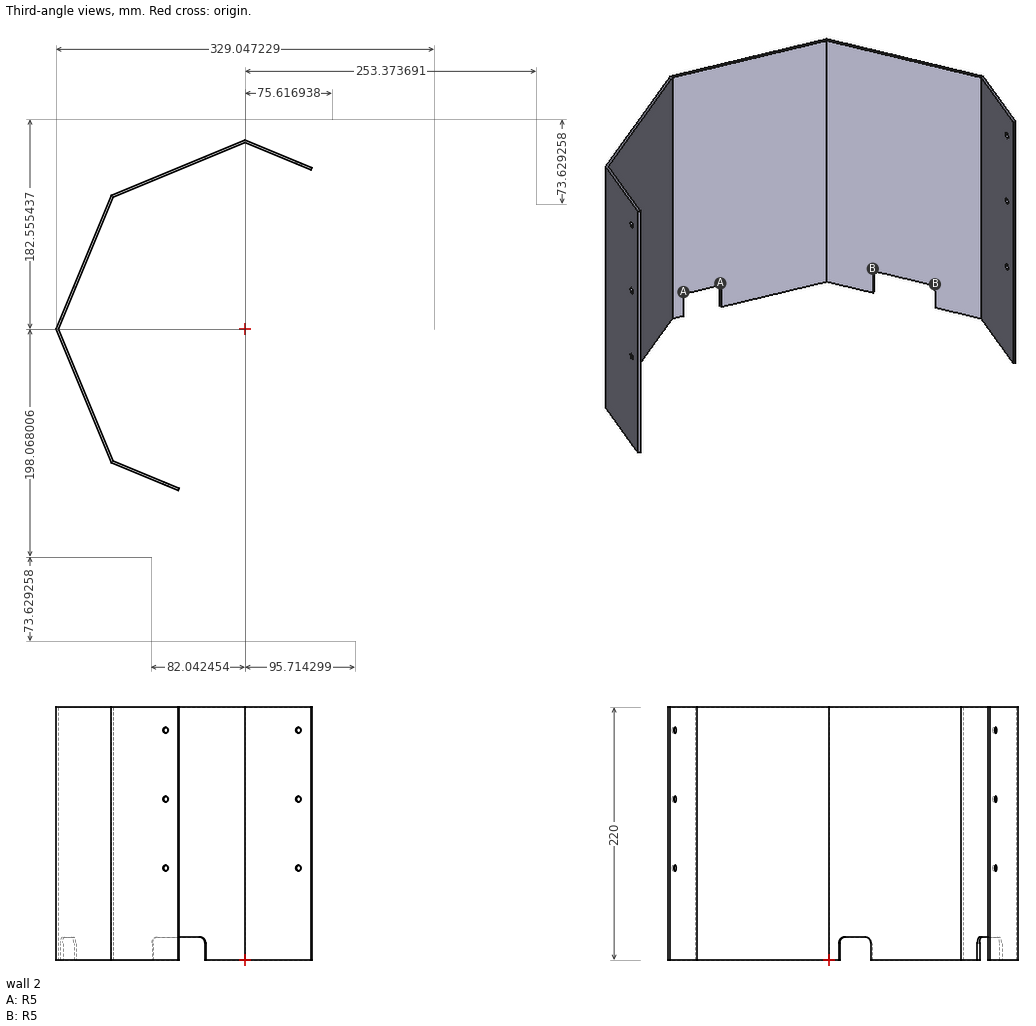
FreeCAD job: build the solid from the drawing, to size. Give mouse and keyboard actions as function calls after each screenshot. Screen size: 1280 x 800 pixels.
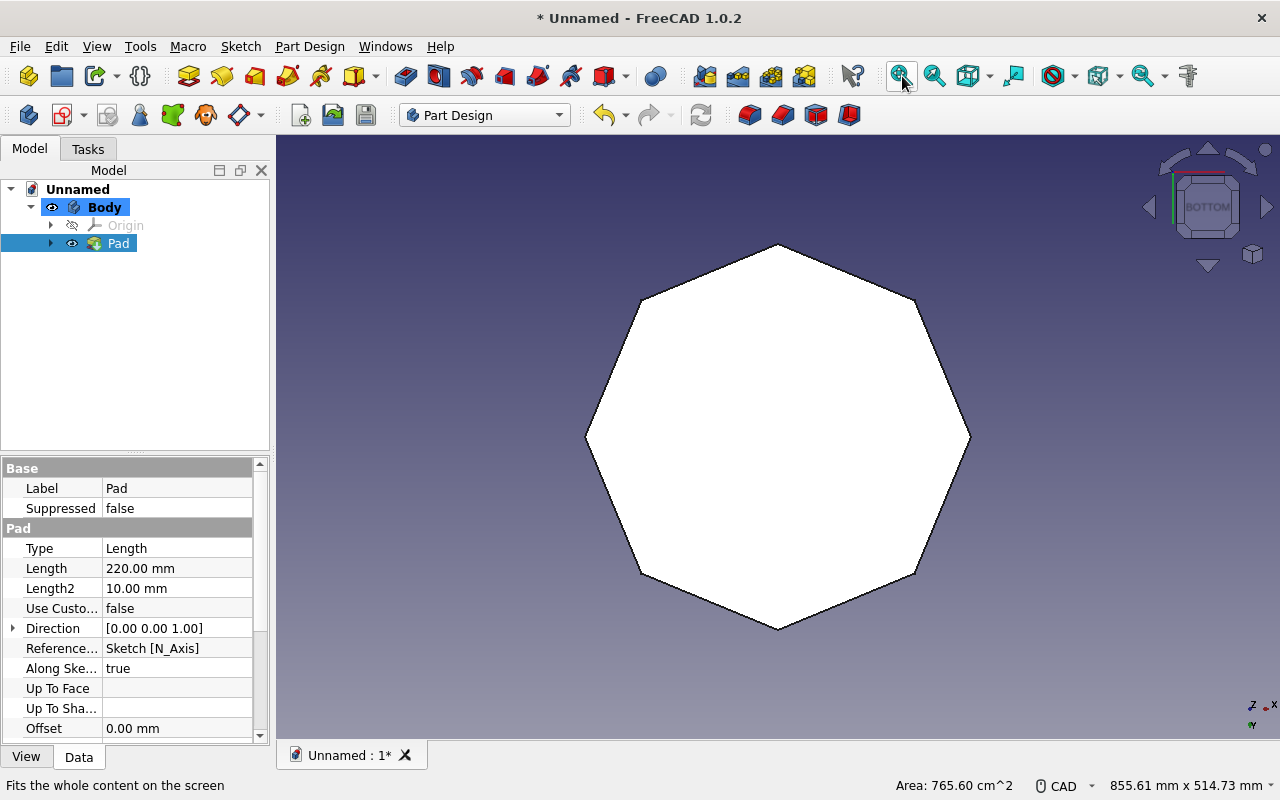
click(778, 436, ctrl)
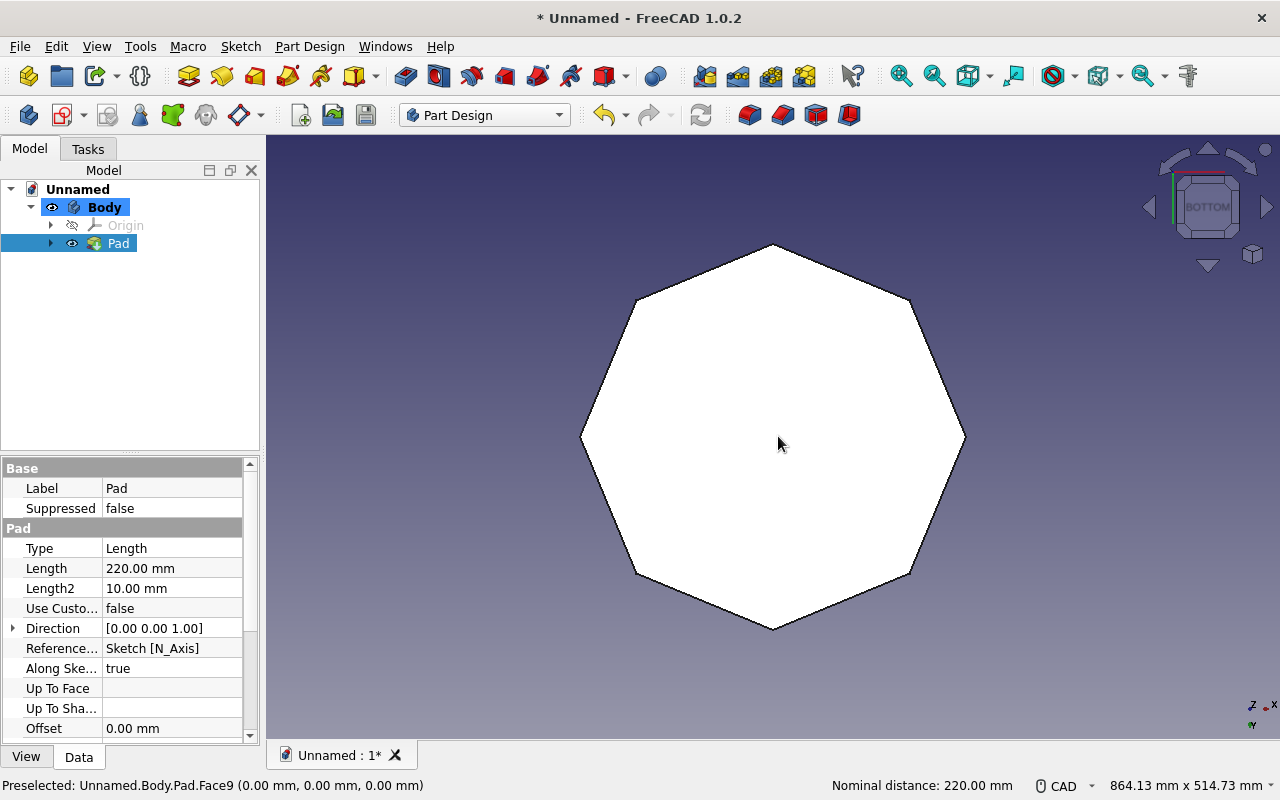
click(849, 116)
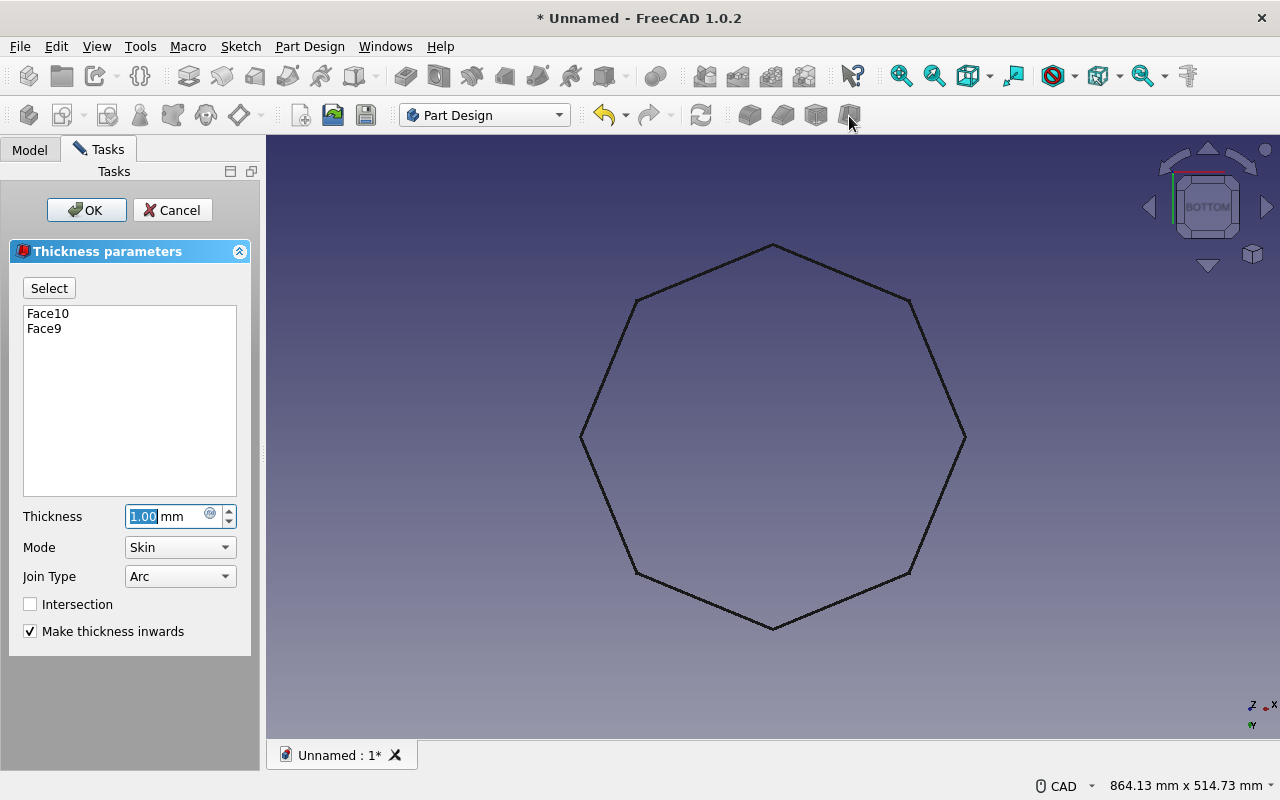
text(2)
key(Tab)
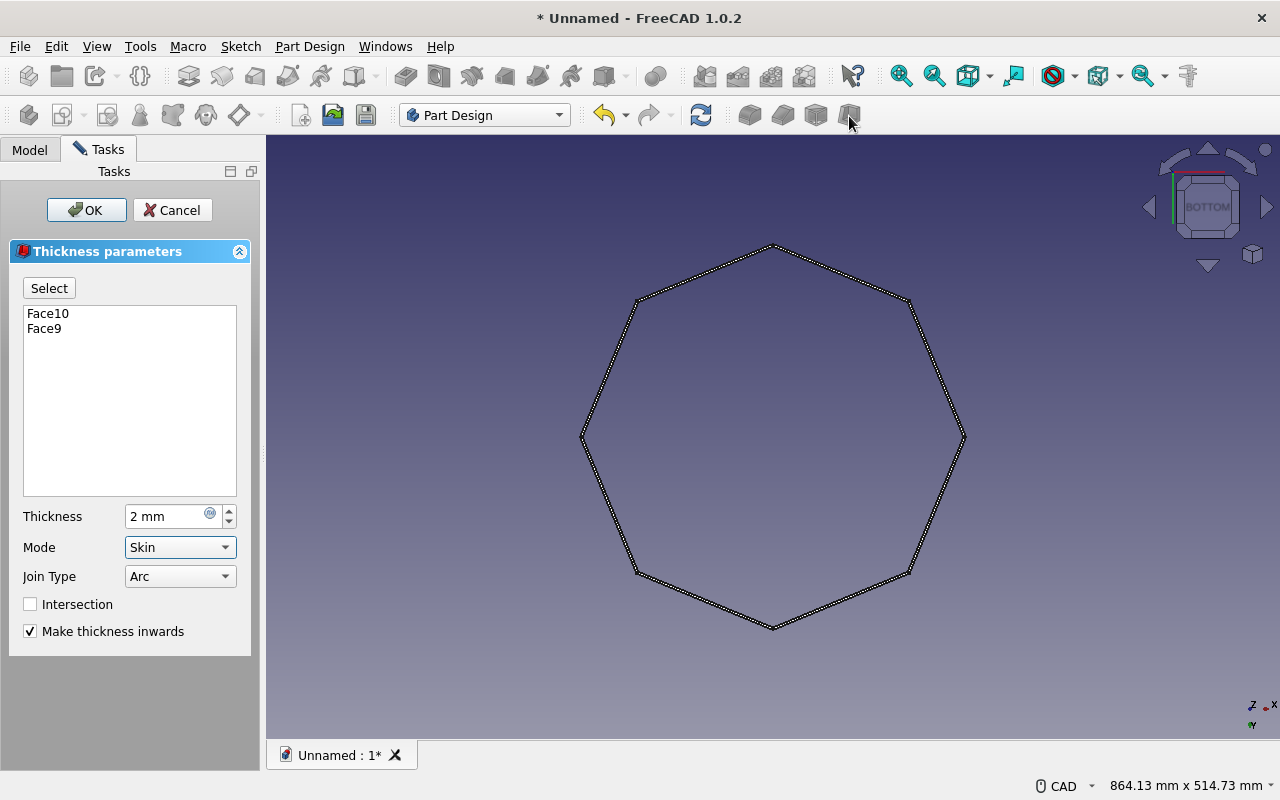
click(181, 576)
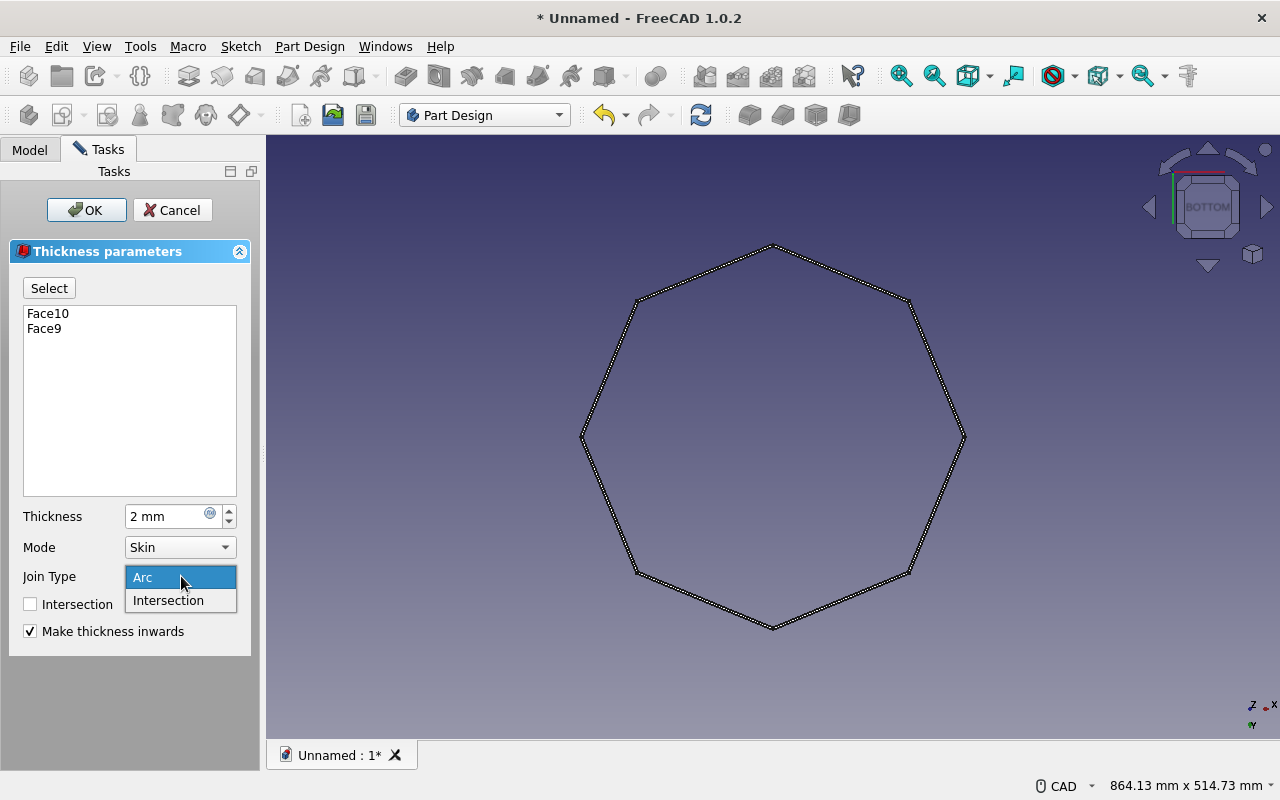
click(179, 600)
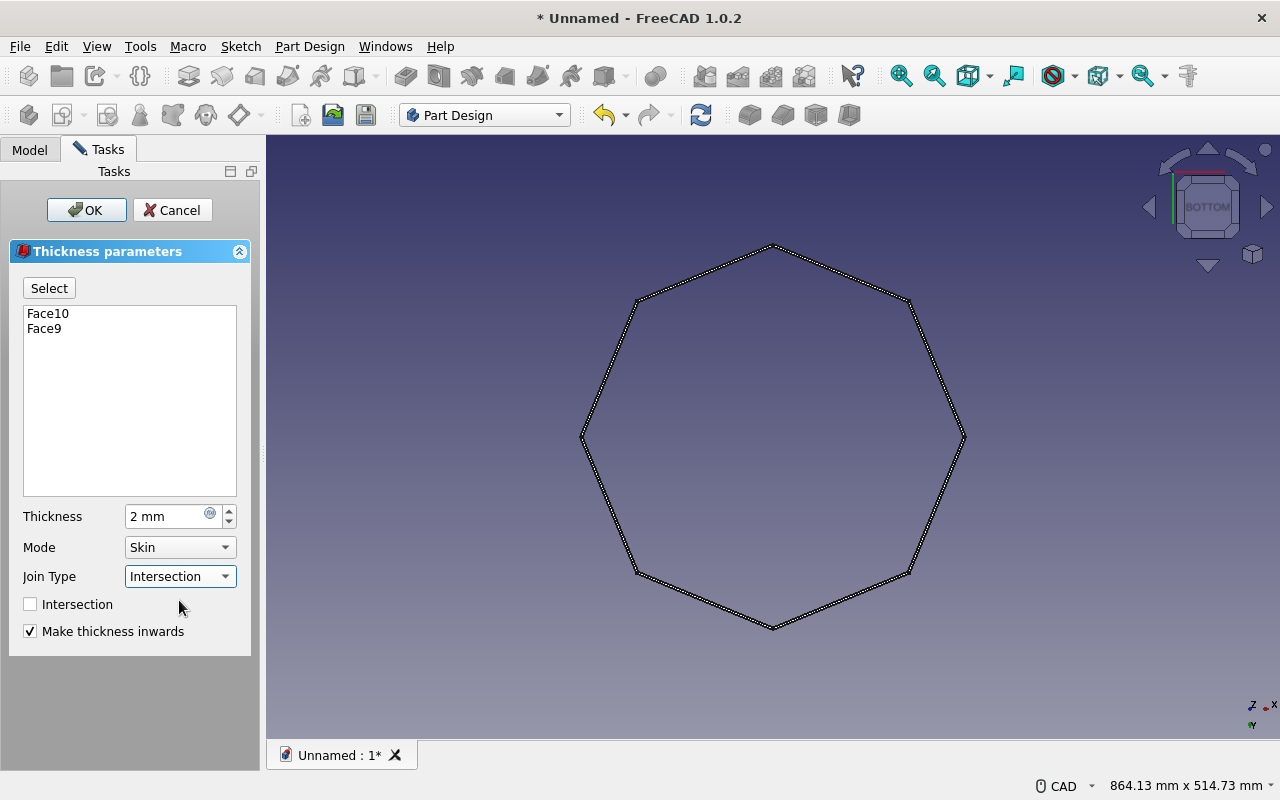
click(87, 210)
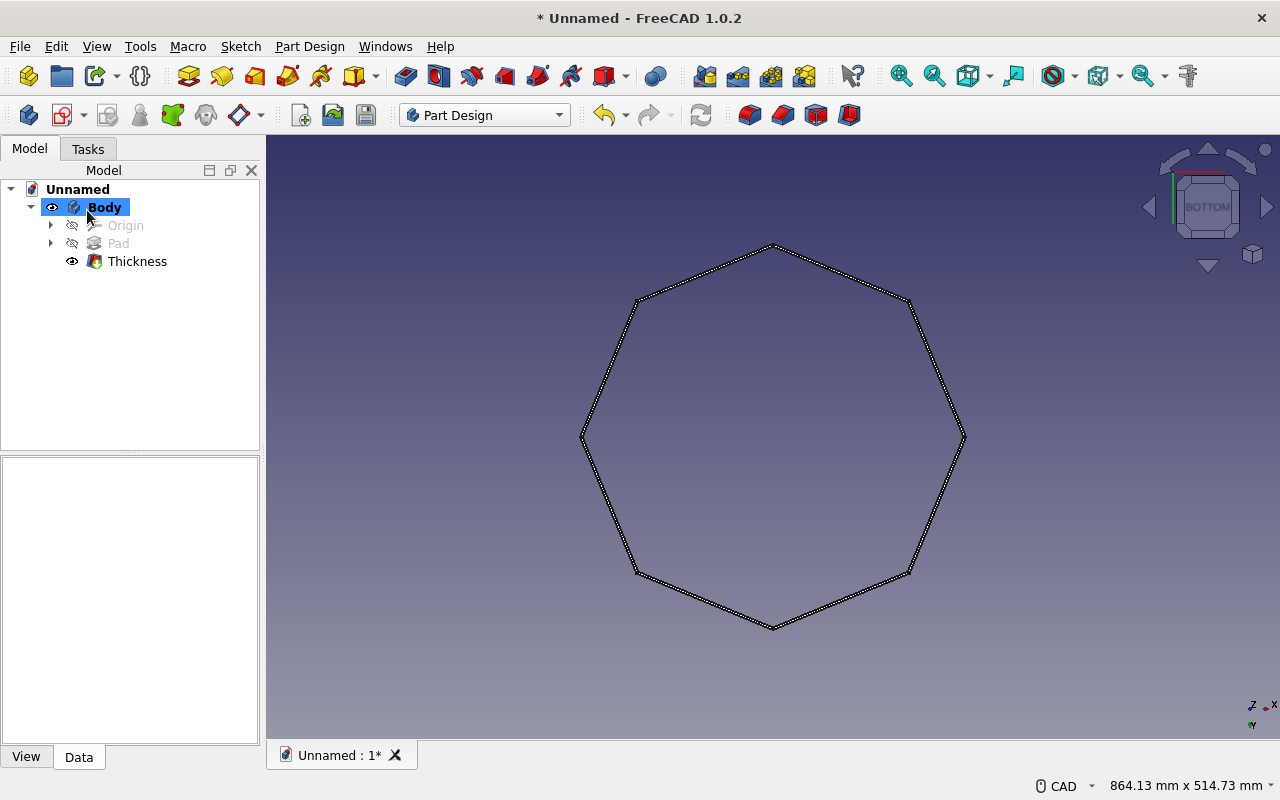
key(0)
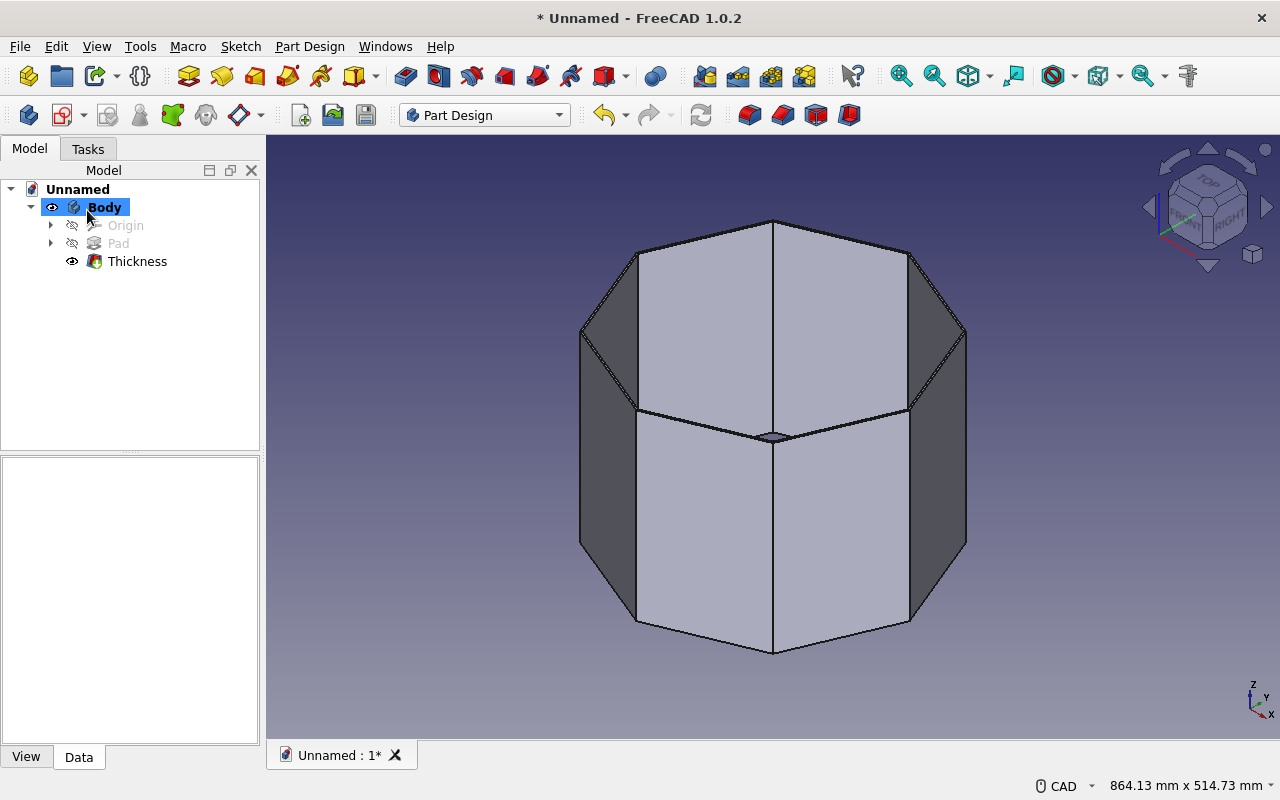
scroll(927, 278, up, 14)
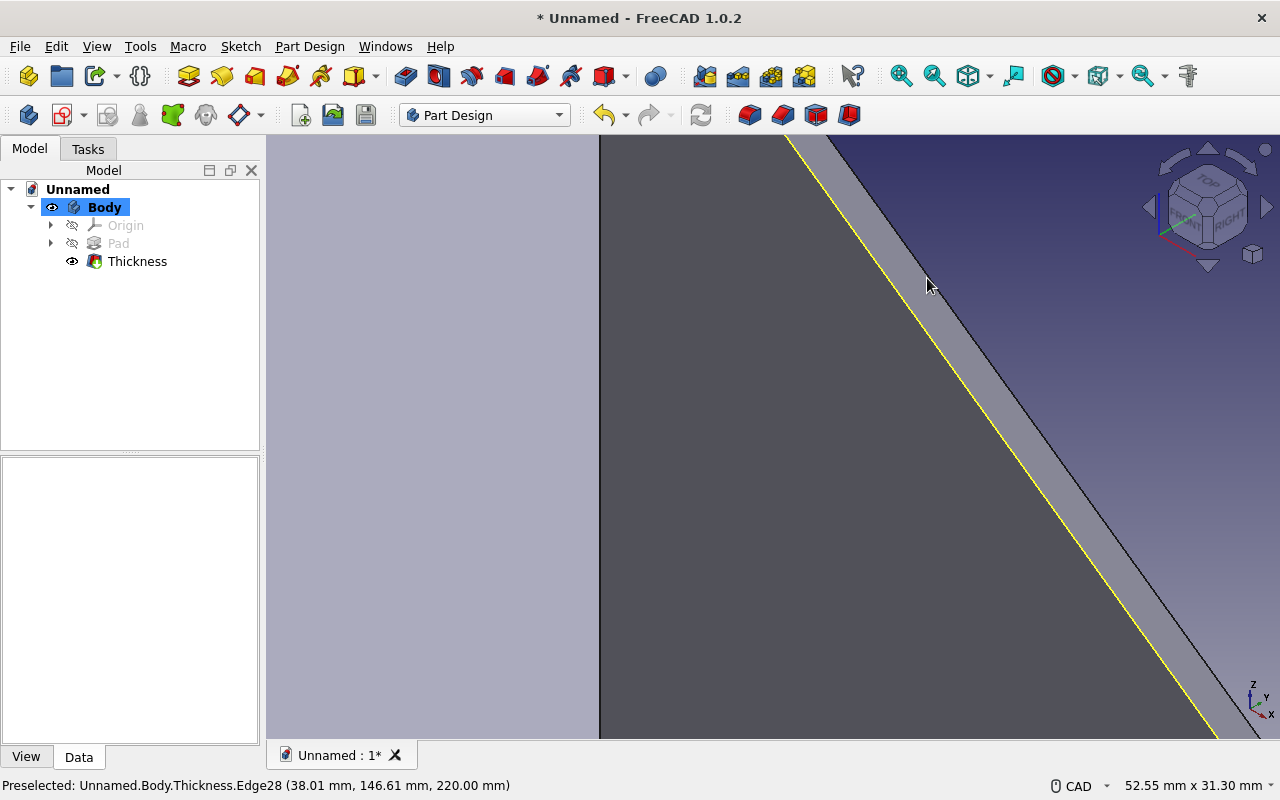
click(916, 297)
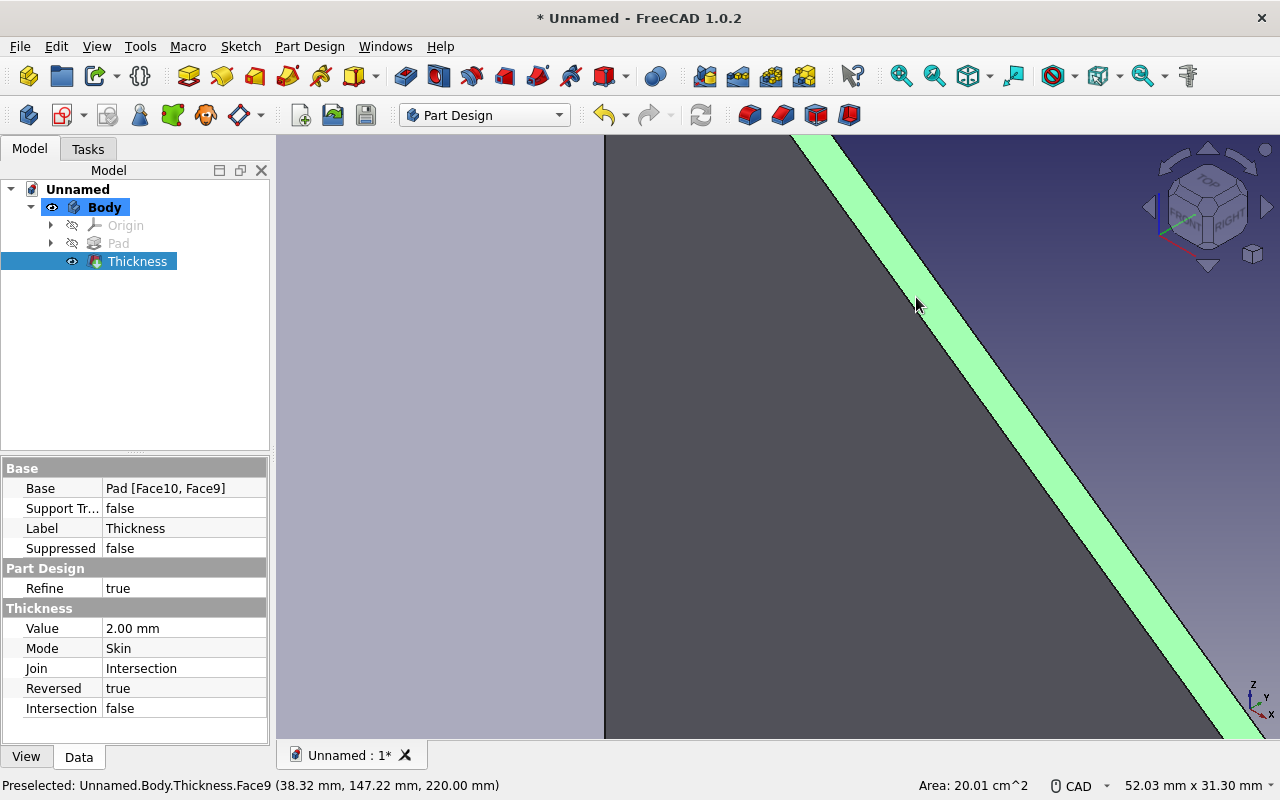
click(62, 116)